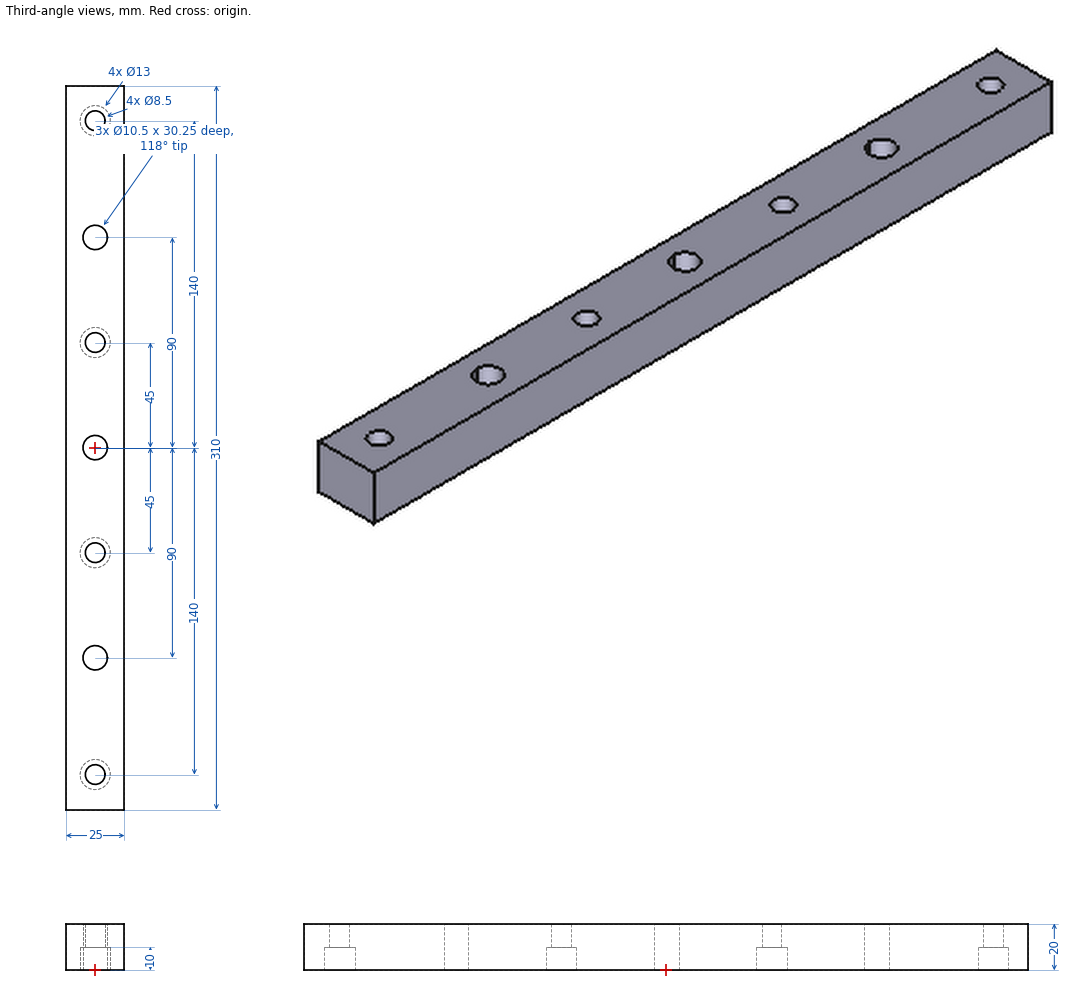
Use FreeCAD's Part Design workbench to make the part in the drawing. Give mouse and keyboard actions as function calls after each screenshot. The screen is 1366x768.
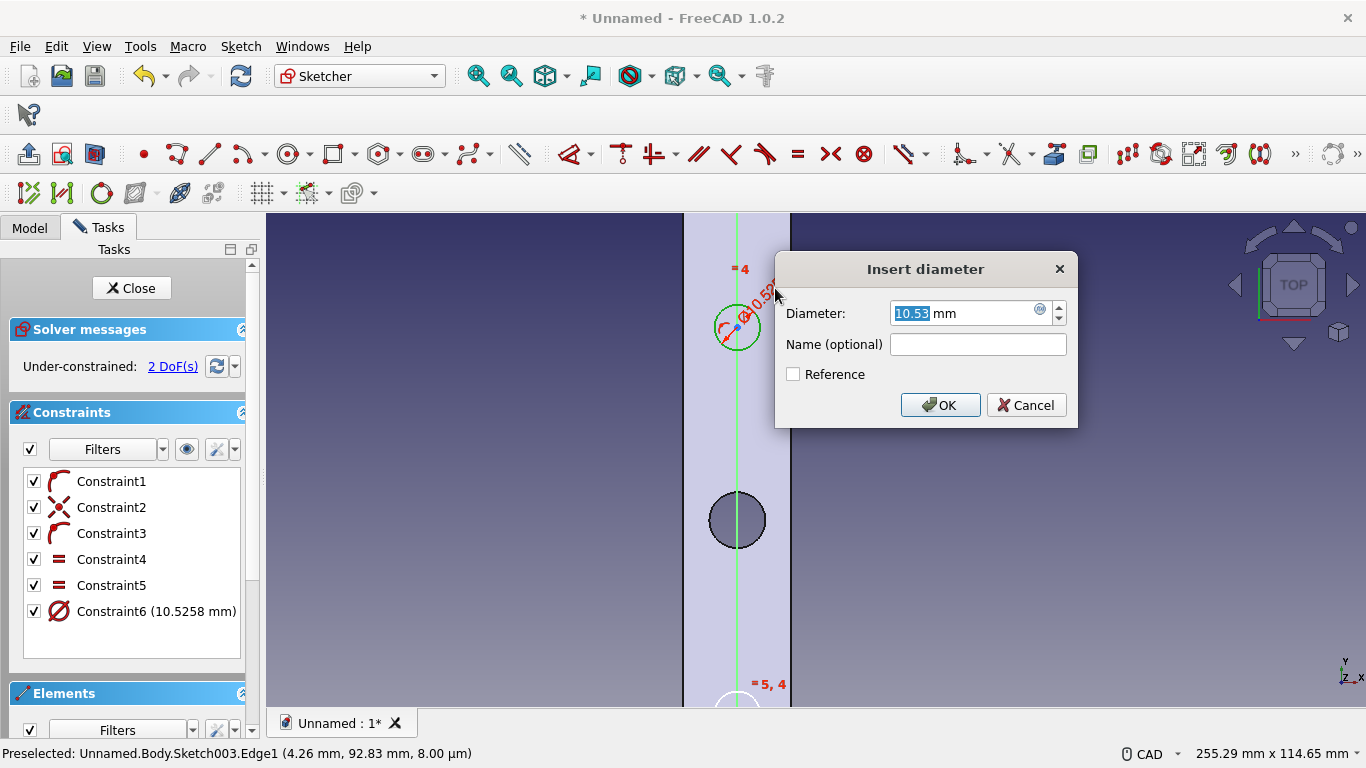
text(10.5)
key(Return)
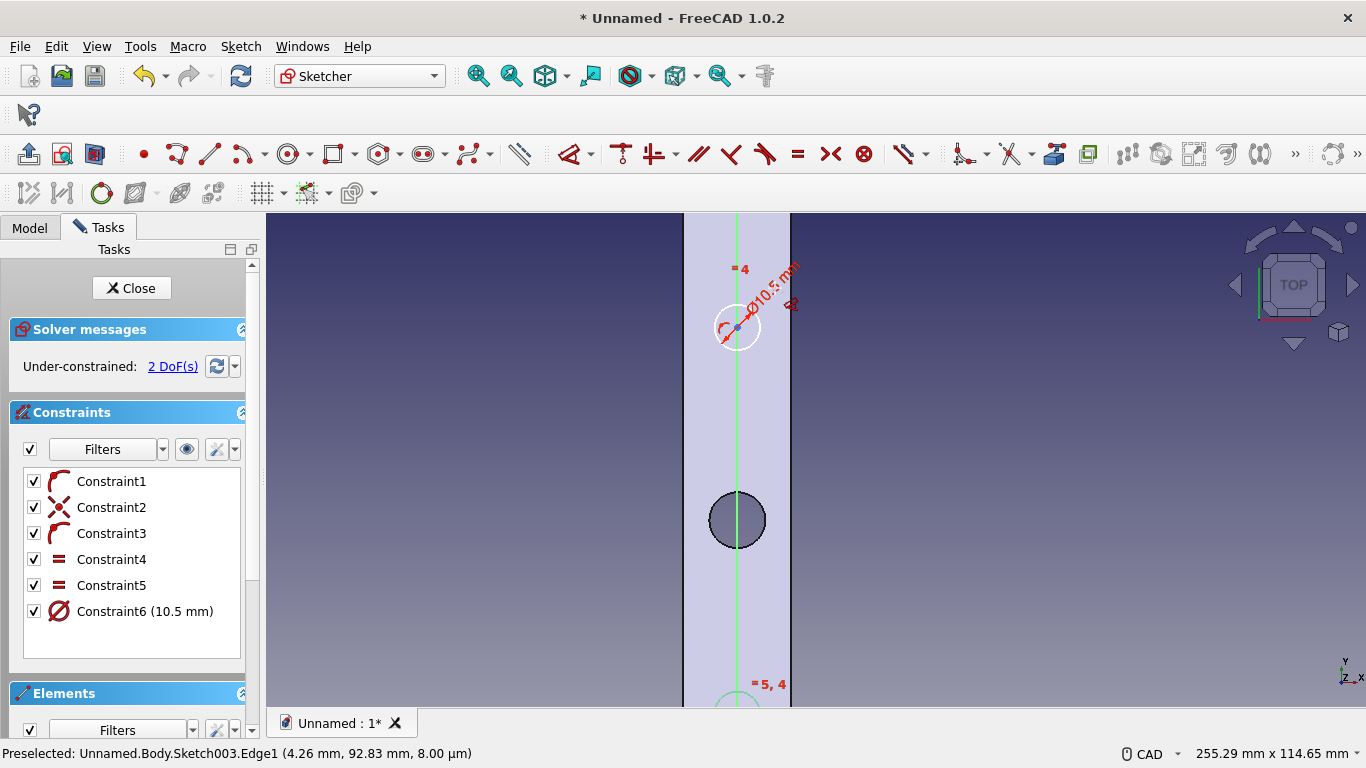
click(737, 327)
click(771, 503)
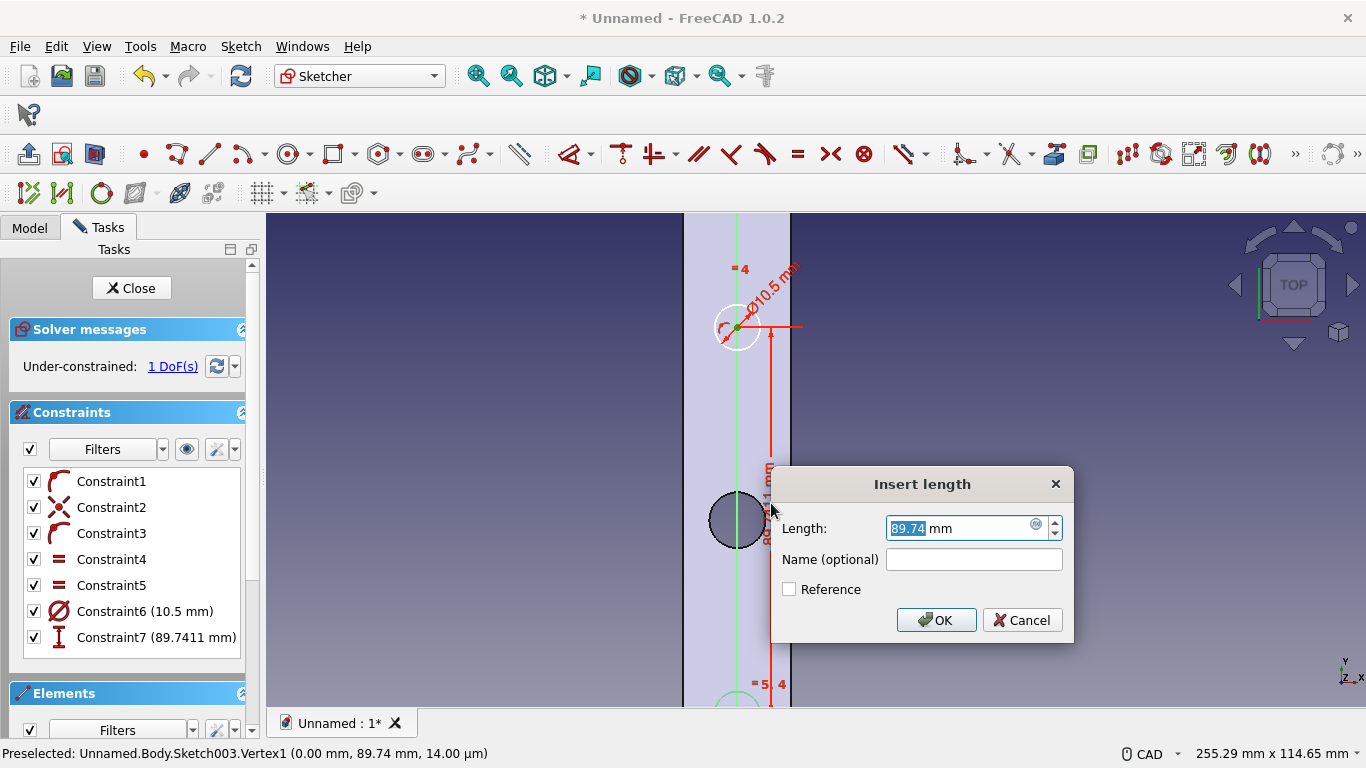
text(90)
key(Return)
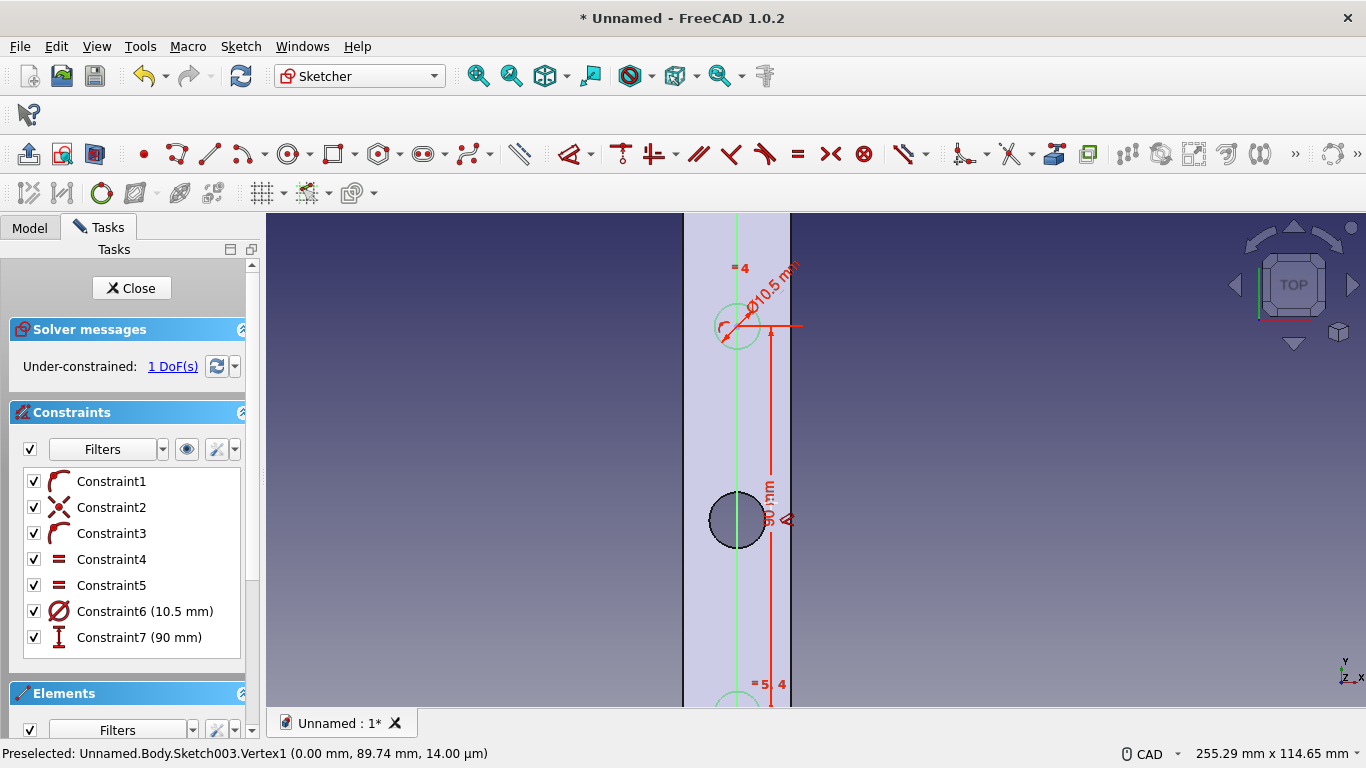
scroll(753, 312, down, 5)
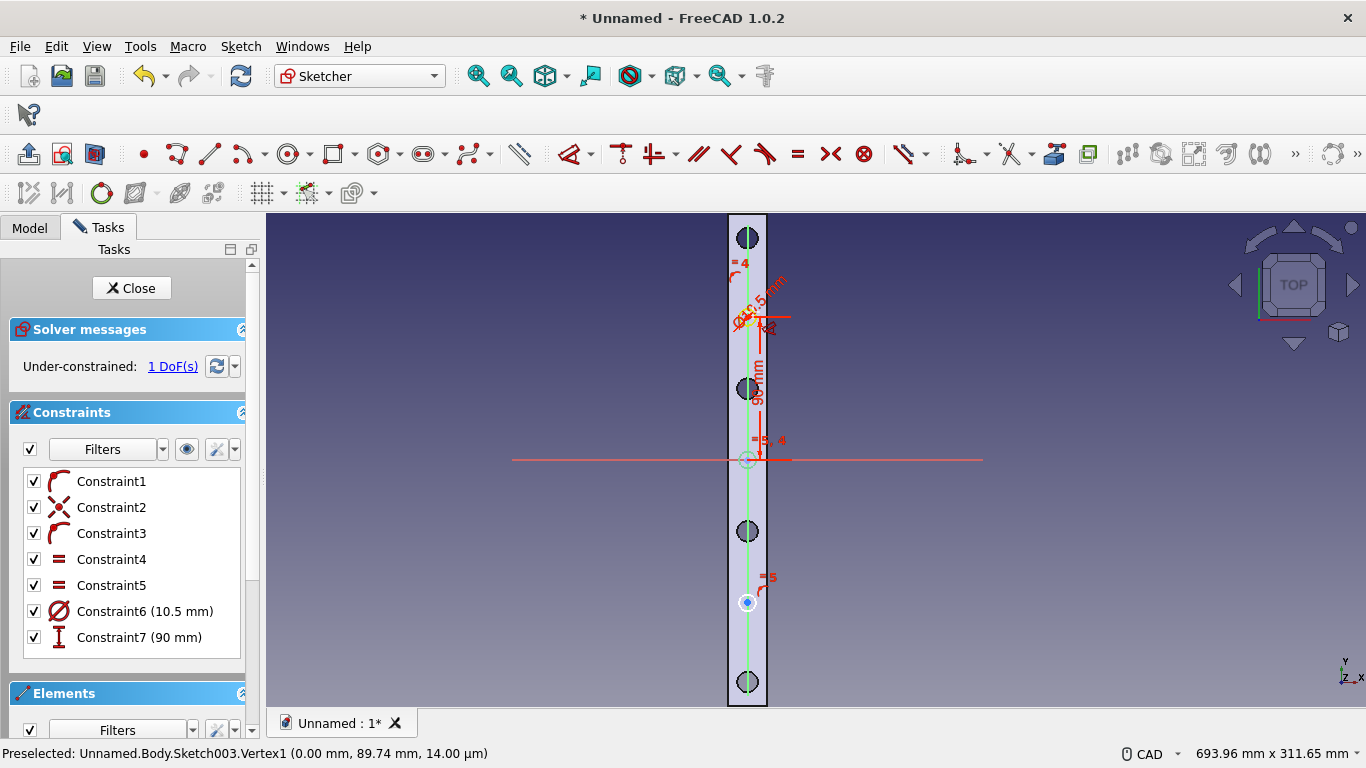
click(748, 603)
click(782, 531)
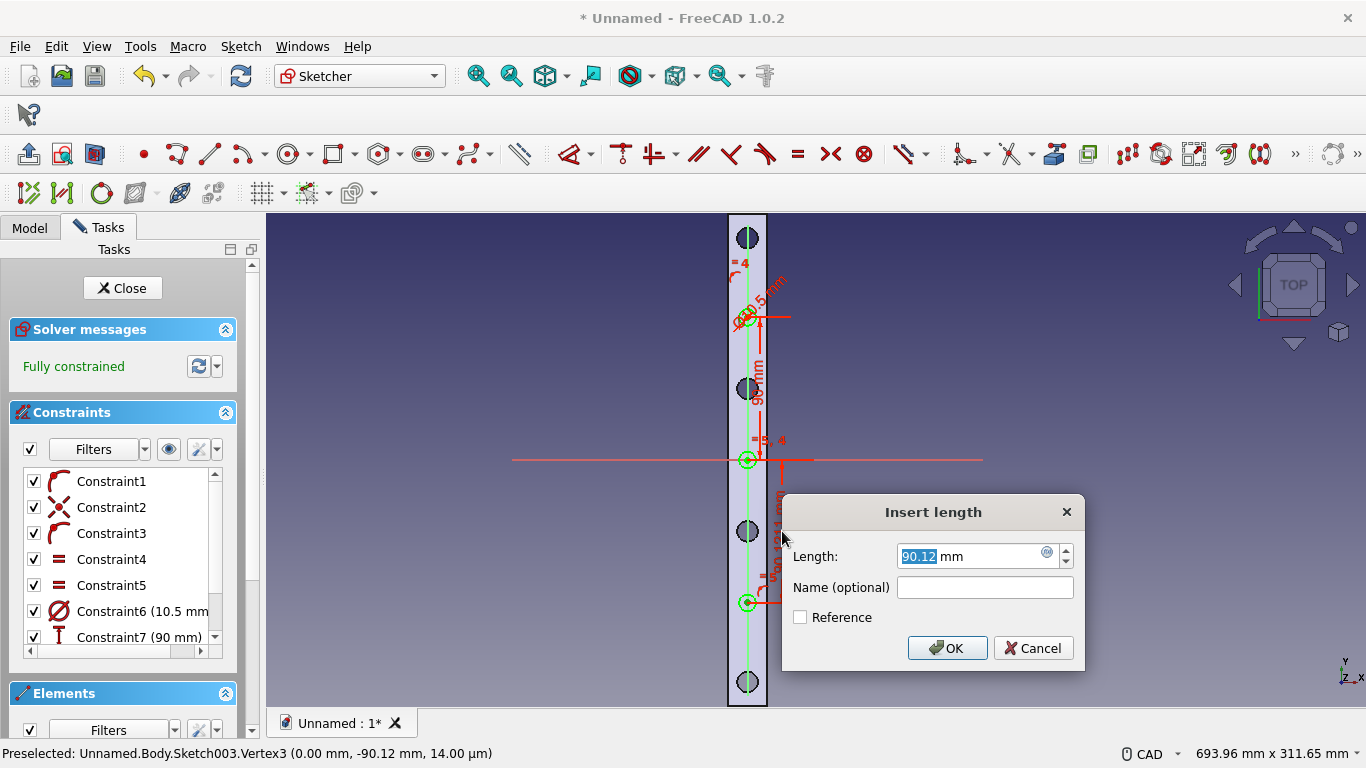
text(90)
key(Return)
key(Escape)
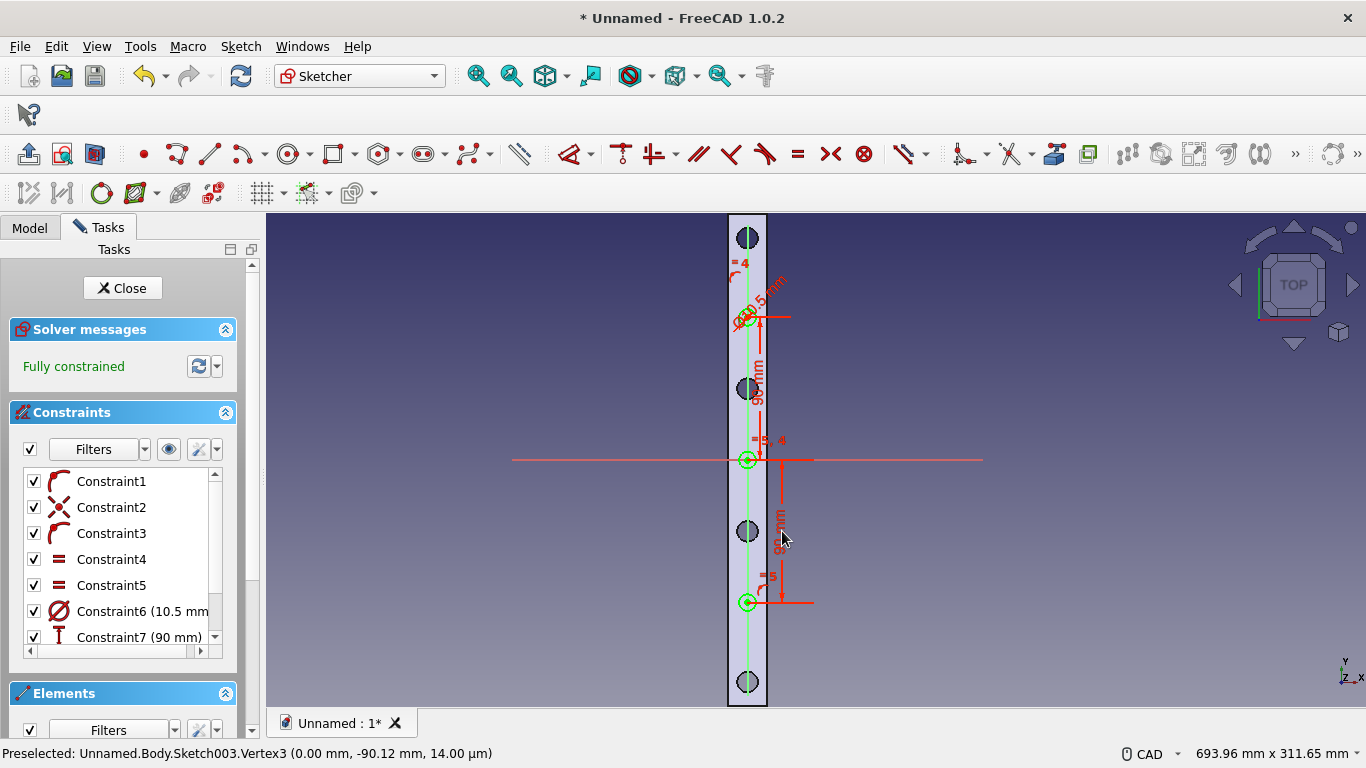
click(123, 288)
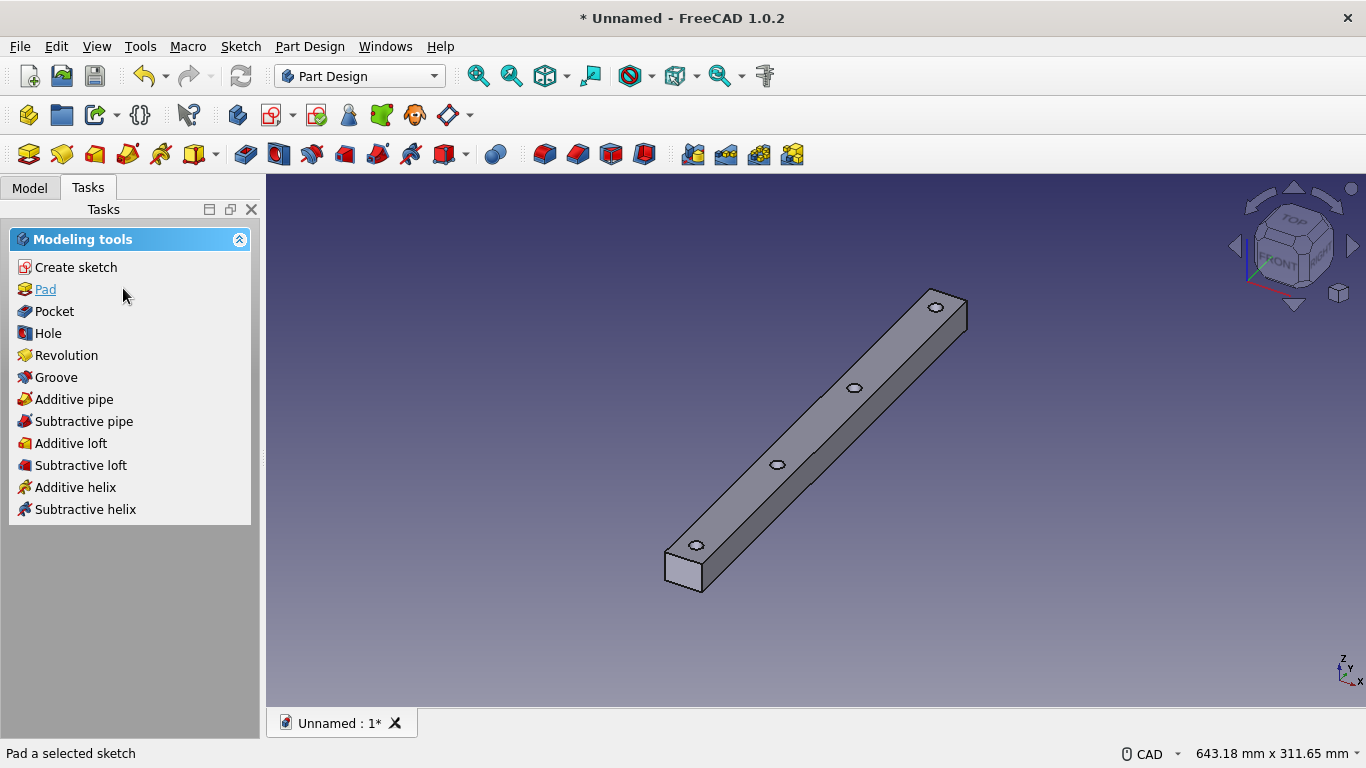
click(279, 154)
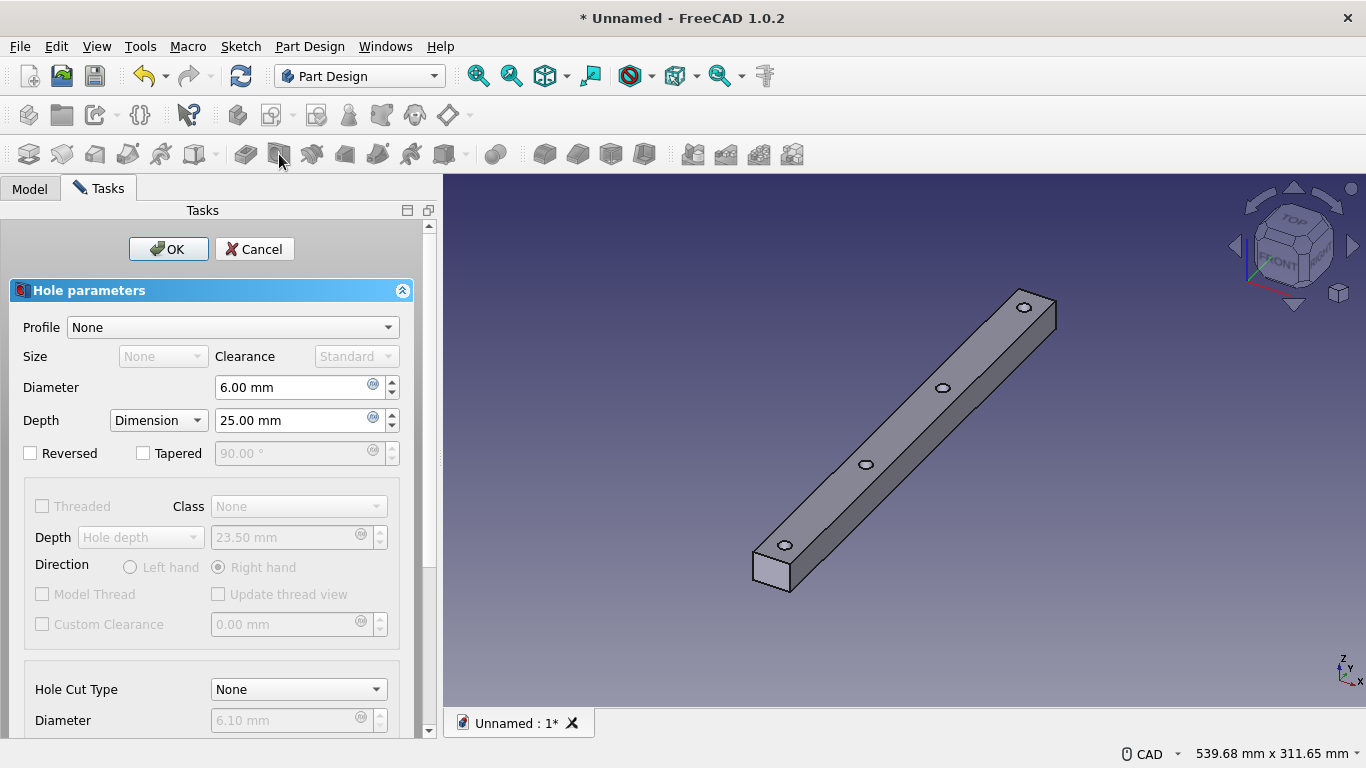
triple_click(300, 388)